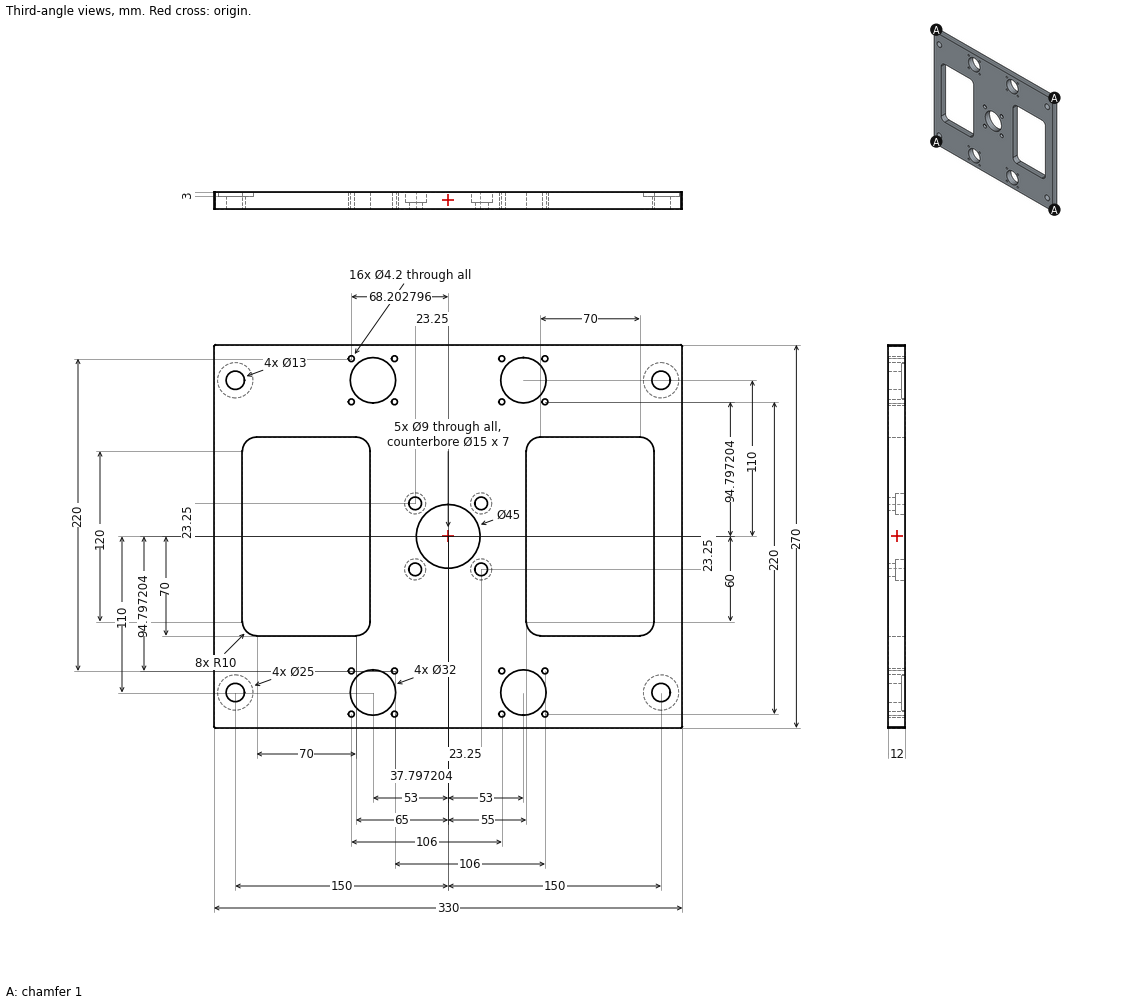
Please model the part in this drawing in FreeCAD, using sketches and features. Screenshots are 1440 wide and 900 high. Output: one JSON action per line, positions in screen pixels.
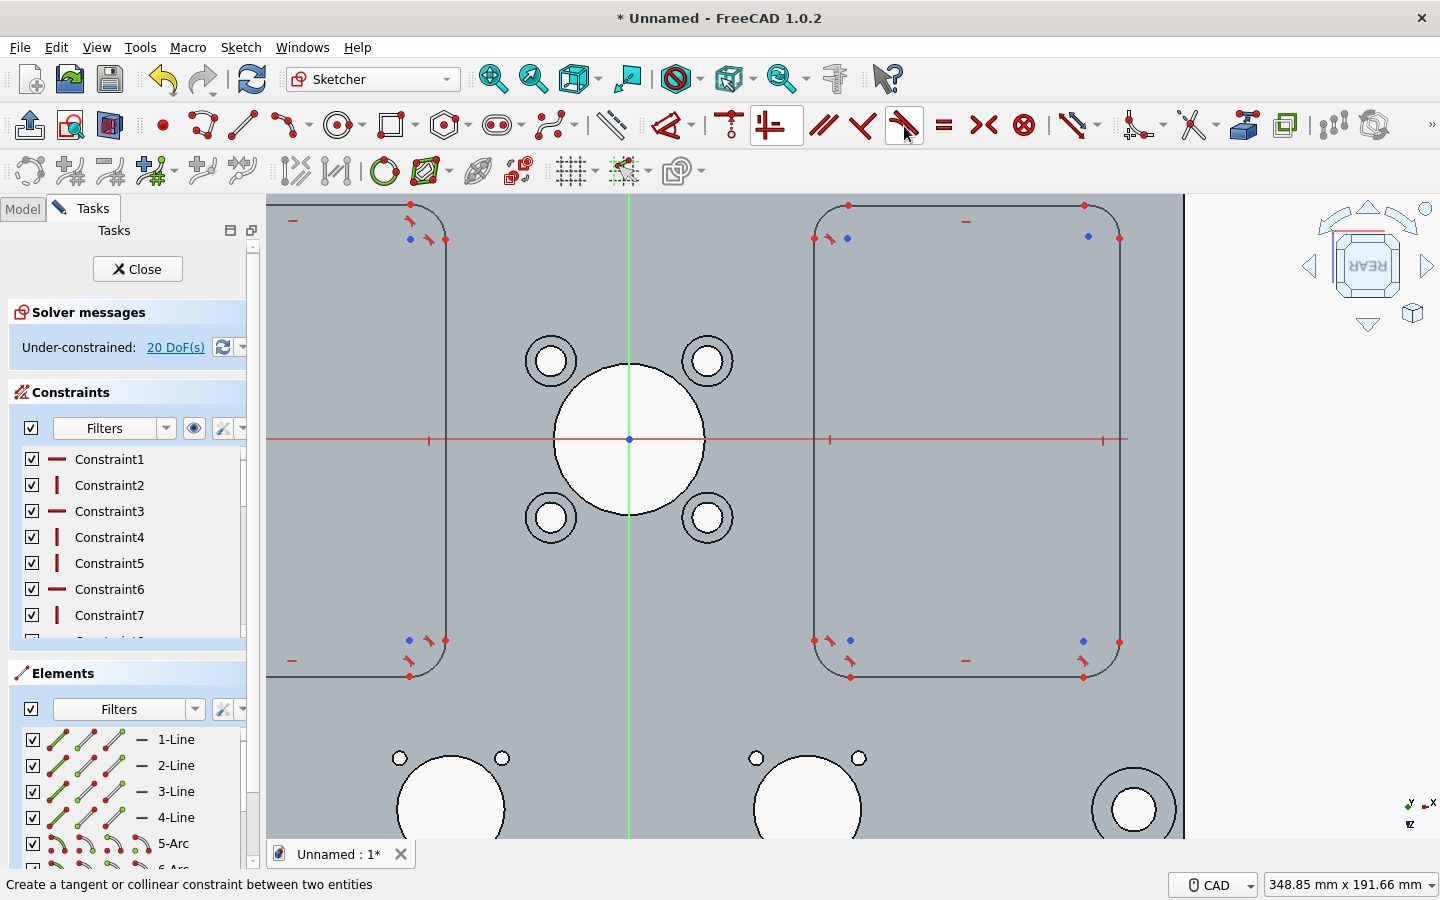
{"action": "left_click", "coordinate": [1120, 522]}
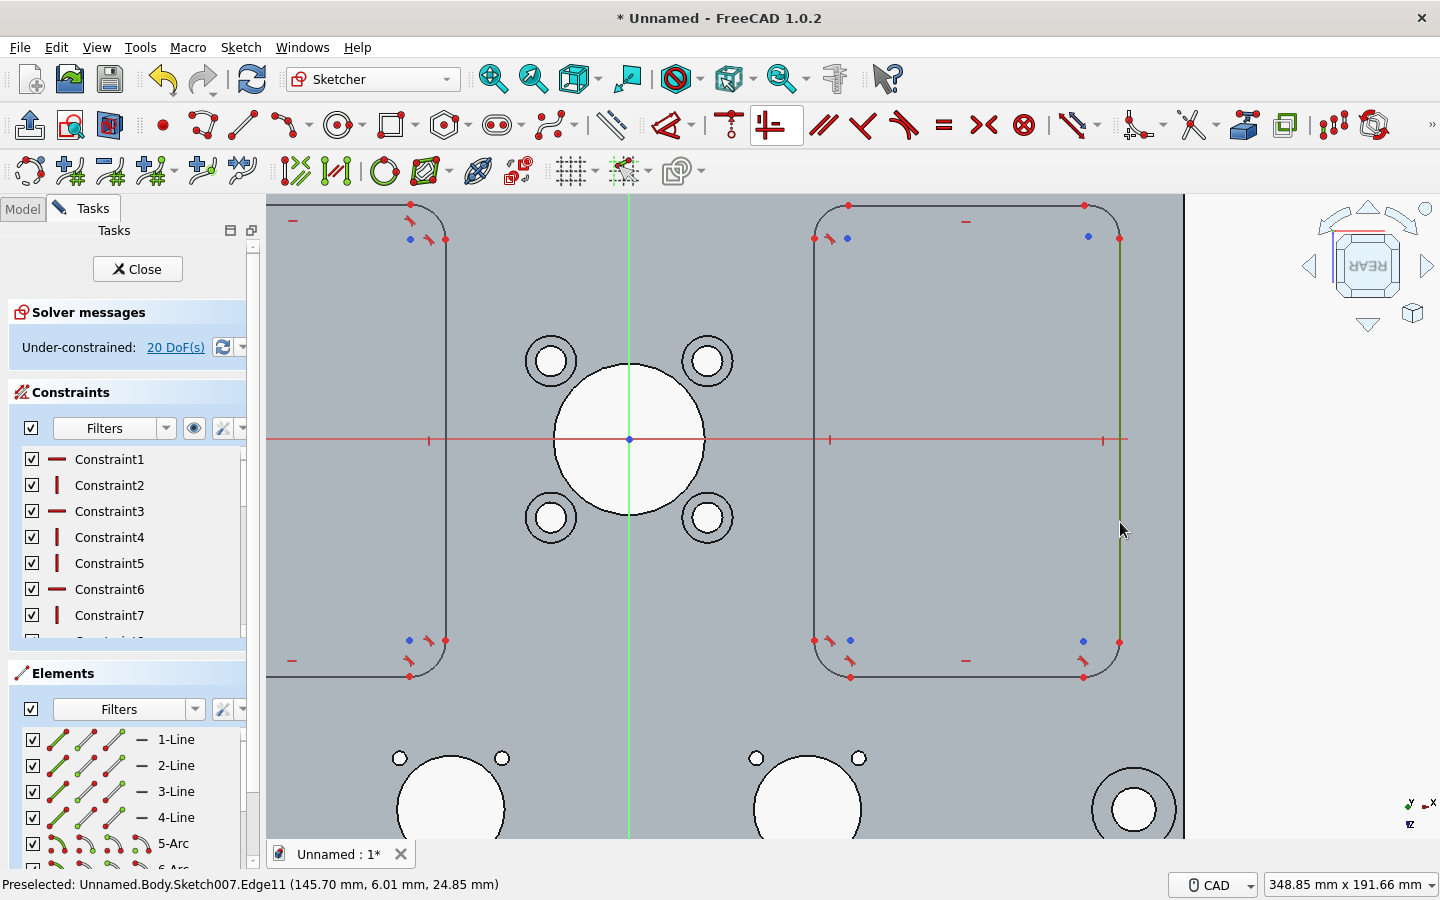
{"action": "left_click", "coordinate": [1099, 673]}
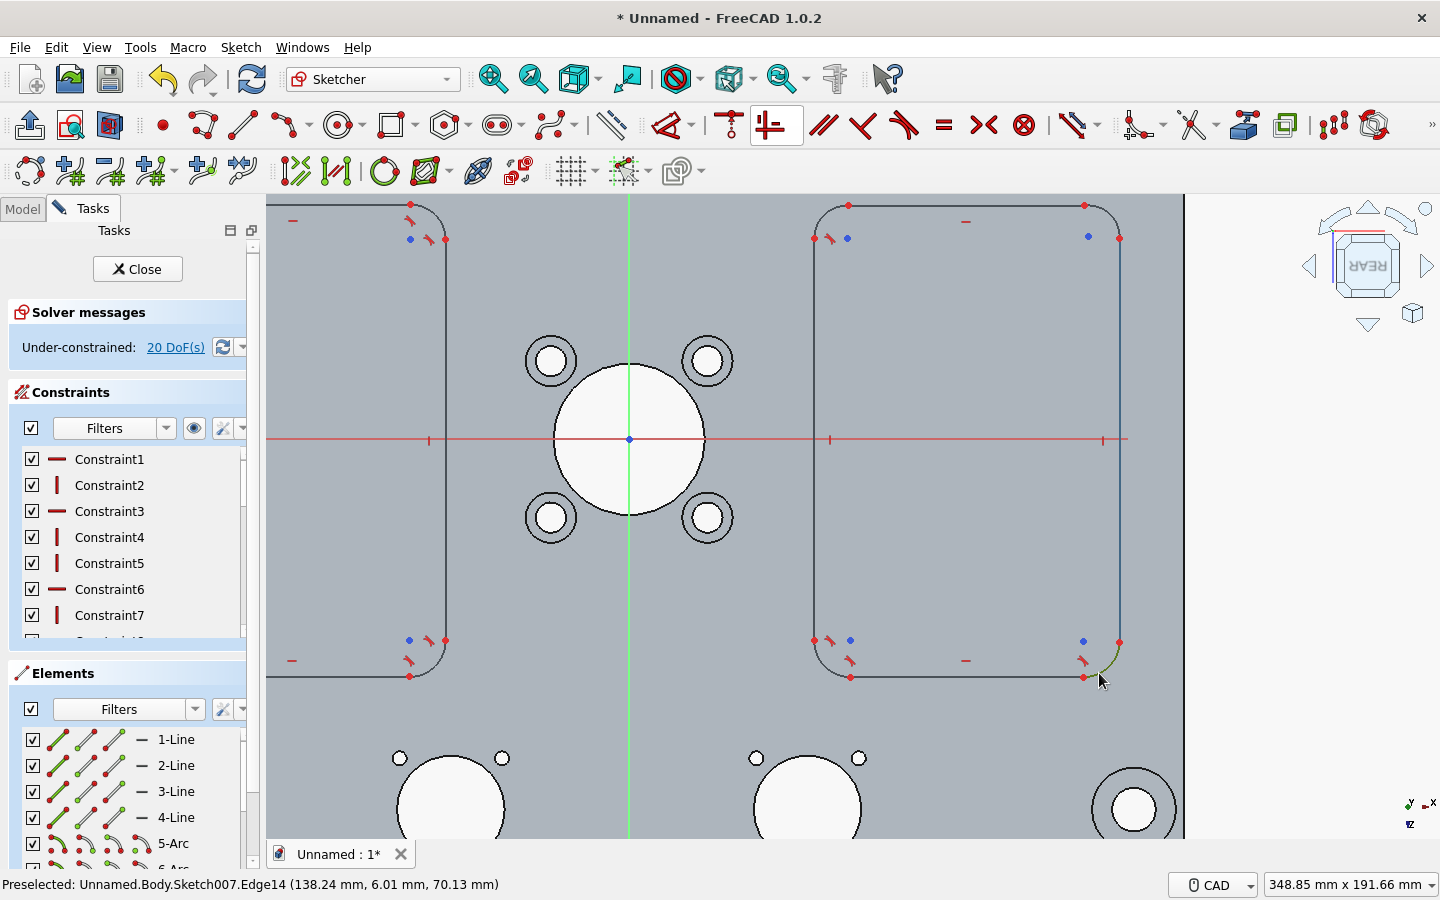
{"action": "left_click", "coordinate": [904, 126]}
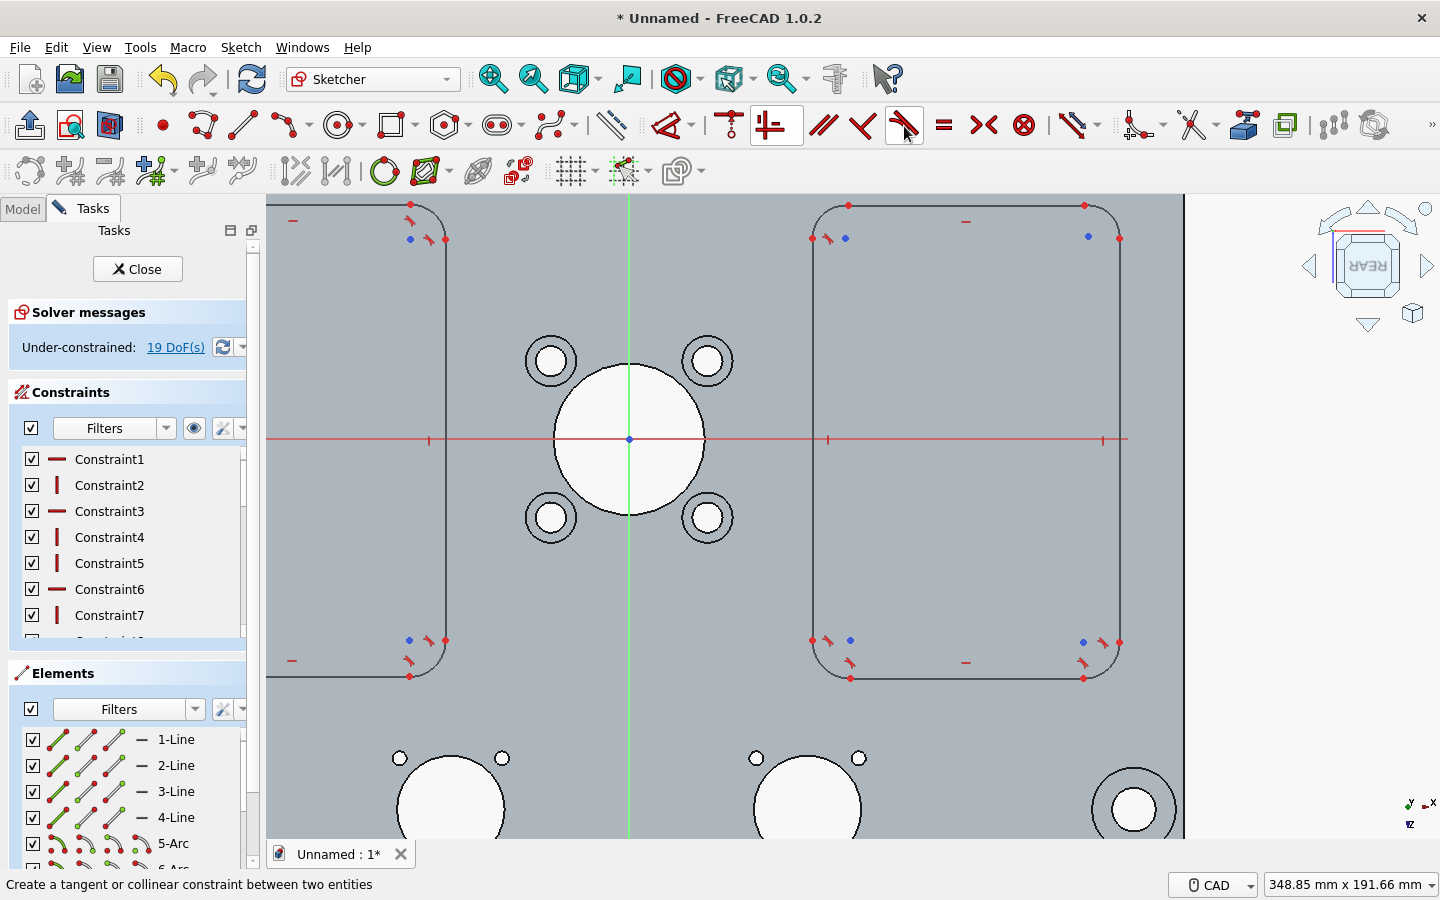
{"action": "left_click", "coordinate": [1120, 522]}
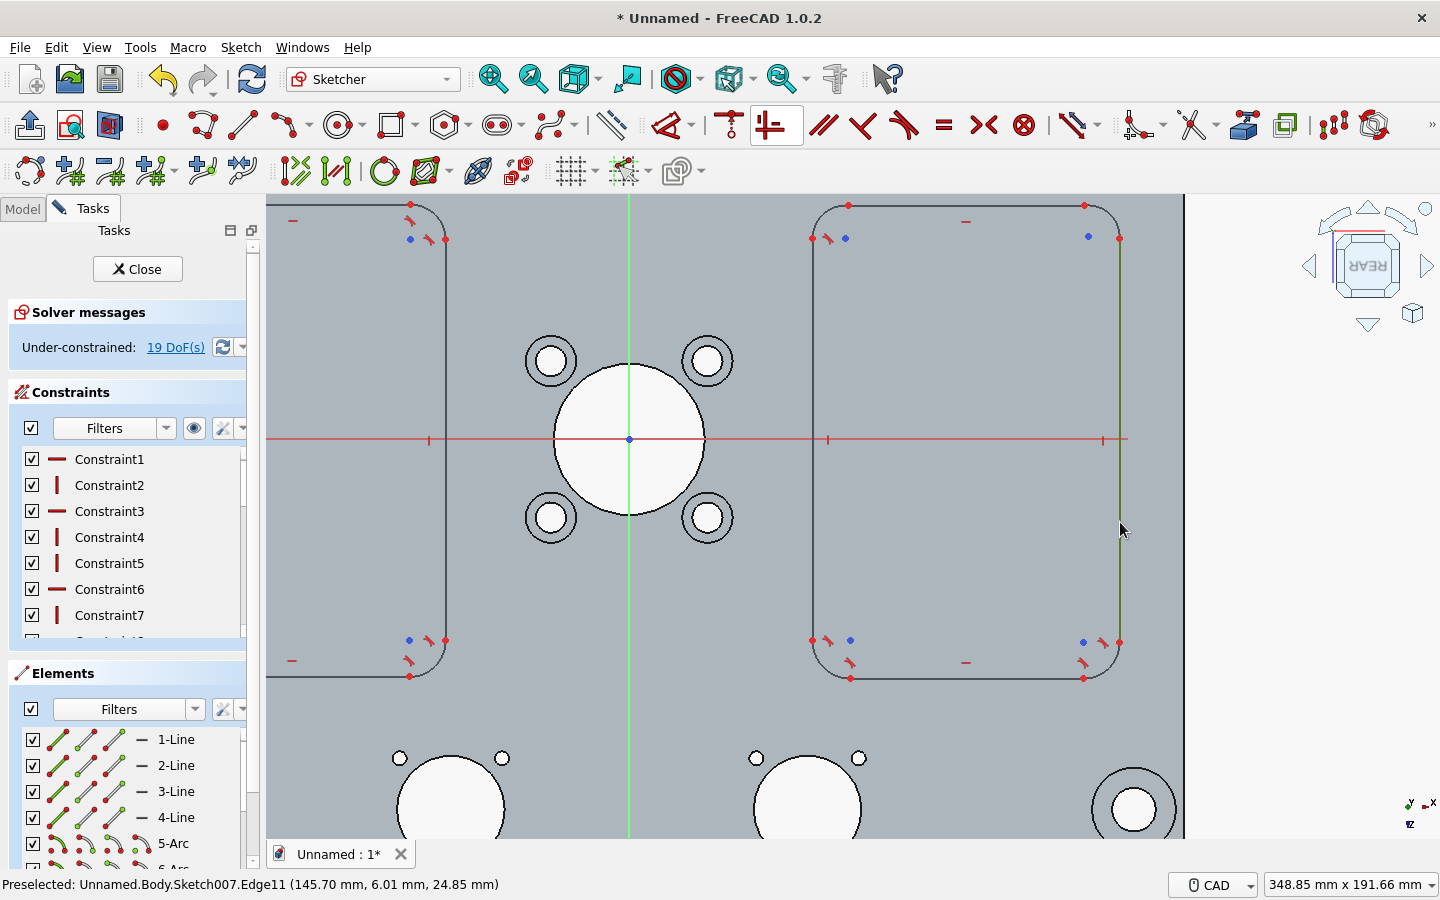
{"action": "left_click", "coordinate": [1116, 223]}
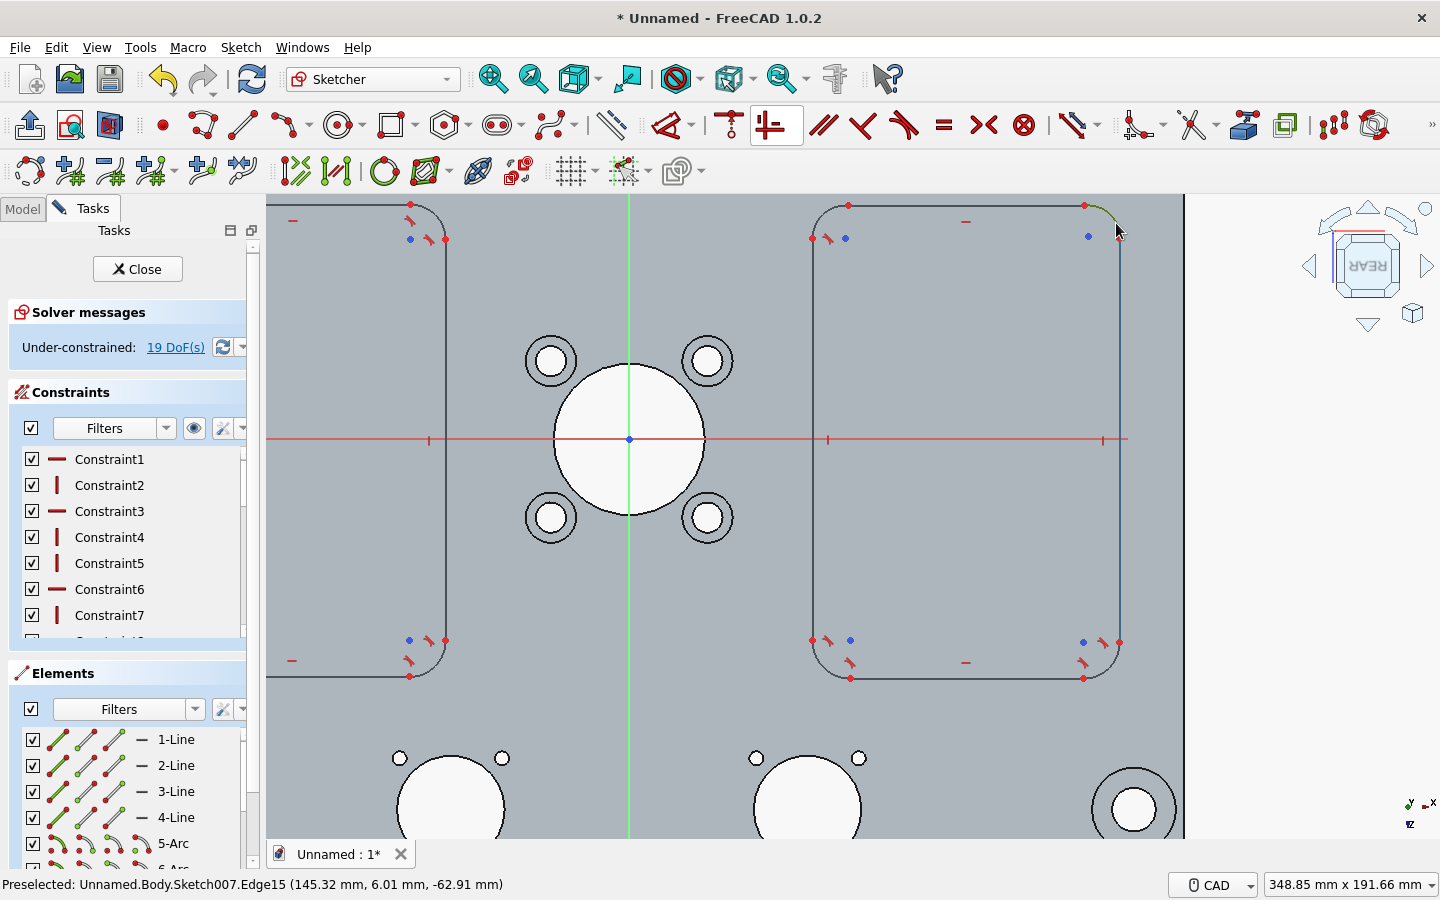
{"action": "left_click", "coordinate": [904, 126]}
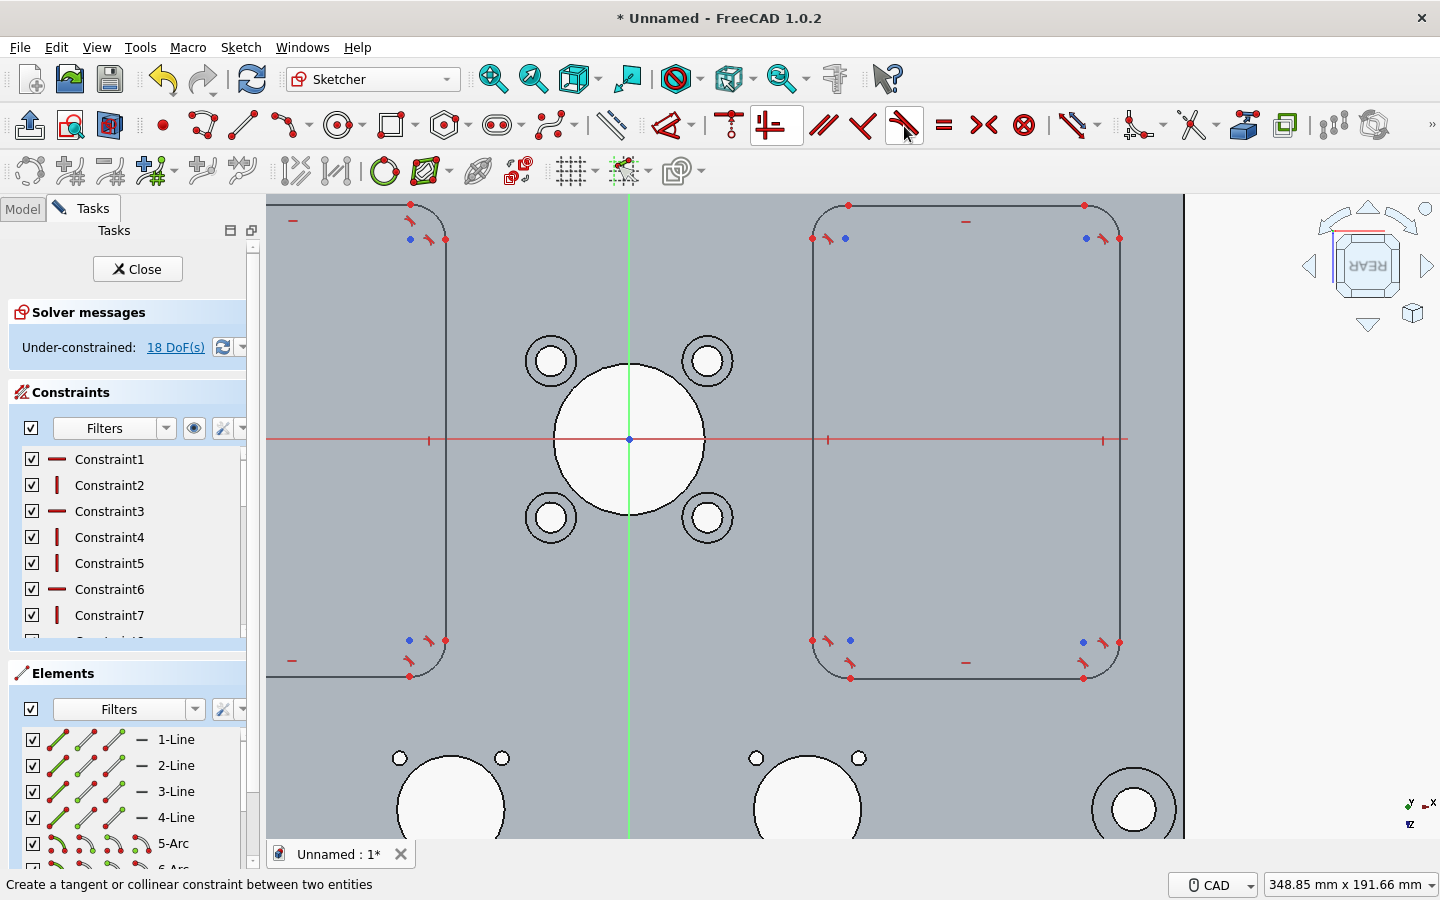
{"action": "scroll", "coordinate": [1100, 673], "scroll_direction": "down", "scroll_amount": 2}